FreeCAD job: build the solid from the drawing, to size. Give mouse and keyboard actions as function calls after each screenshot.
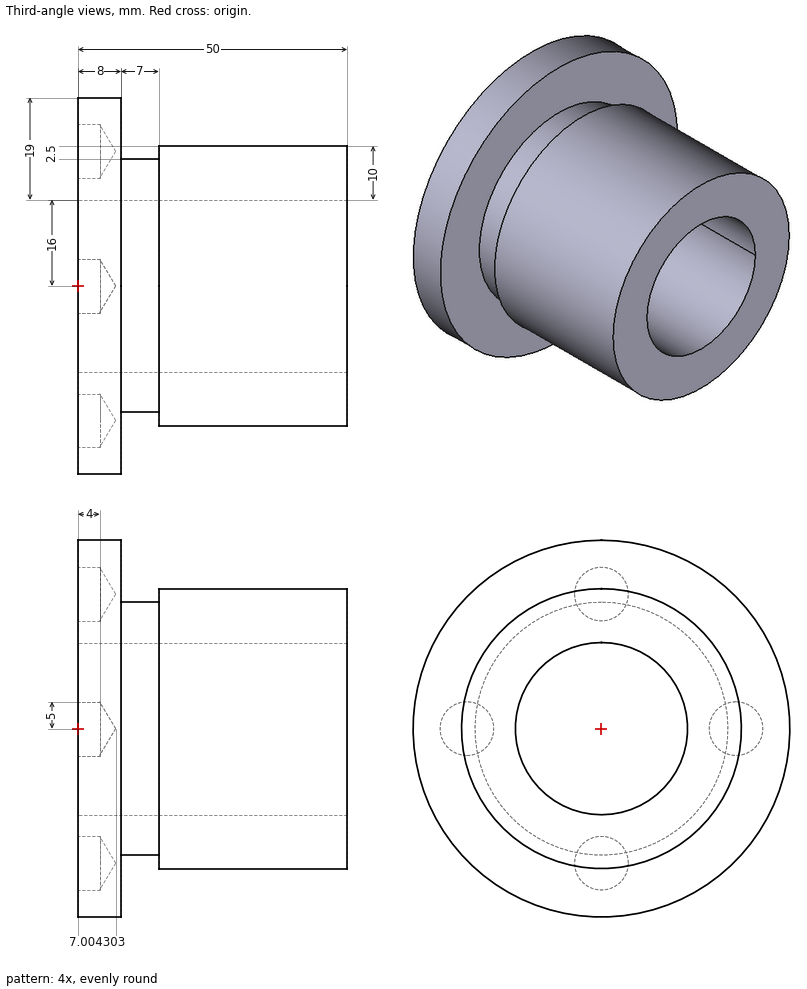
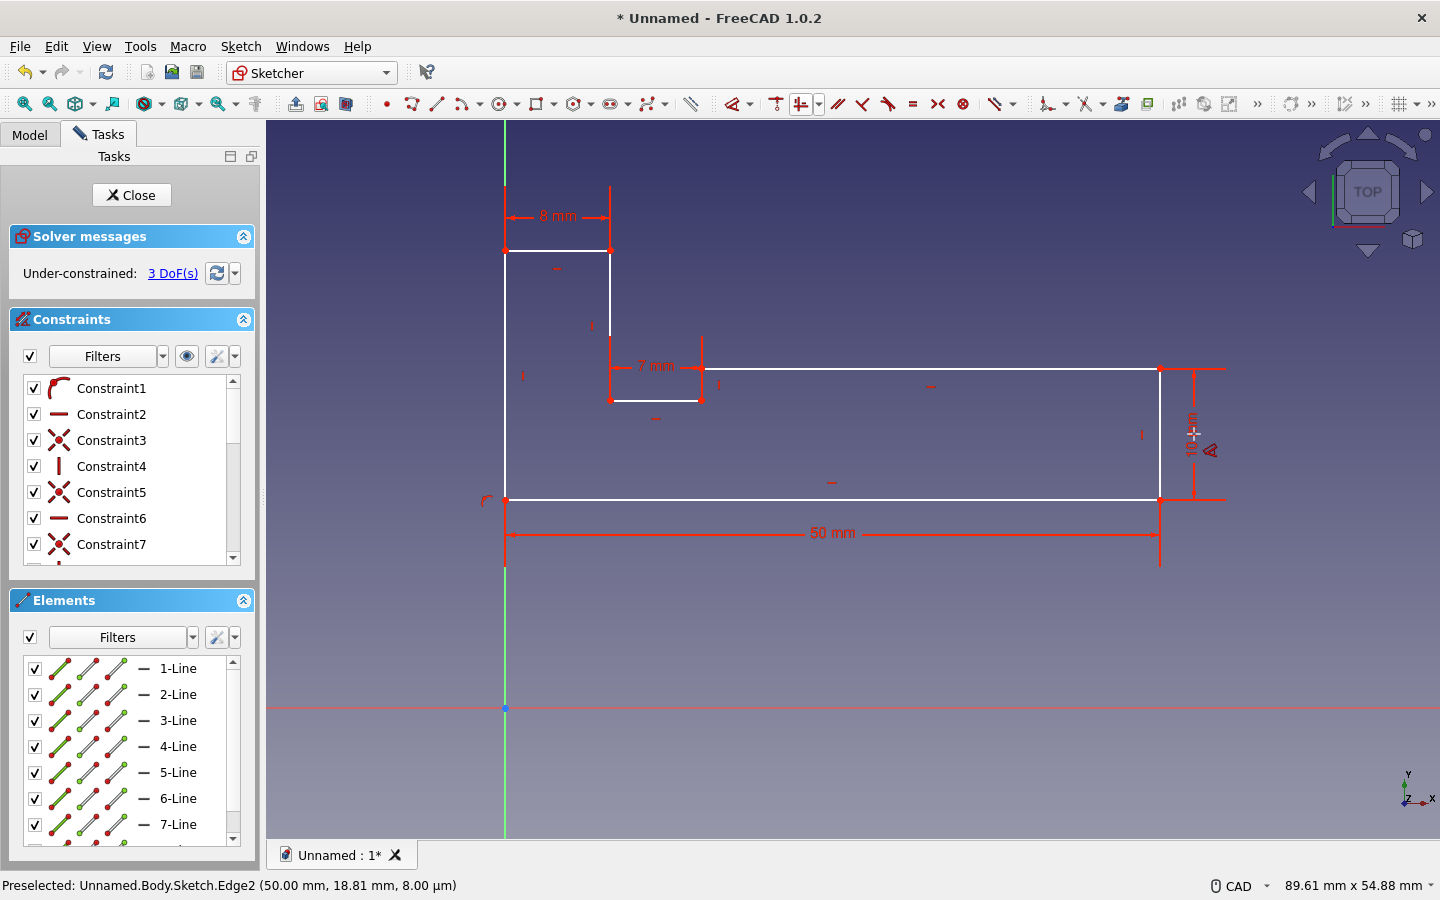
click(505, 326)
click(471, 376)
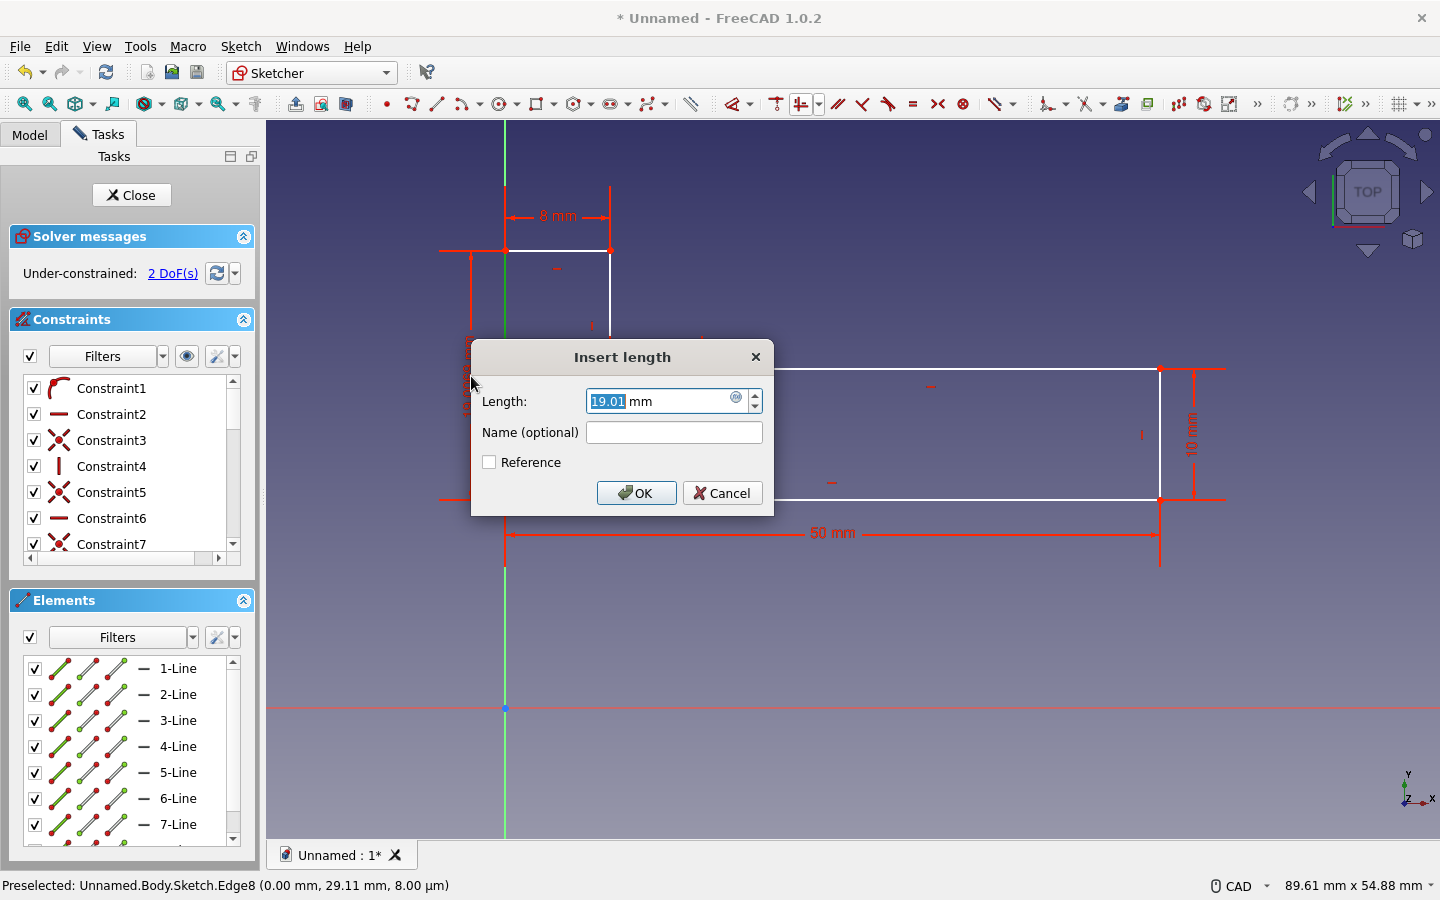
text(19)
key(Return)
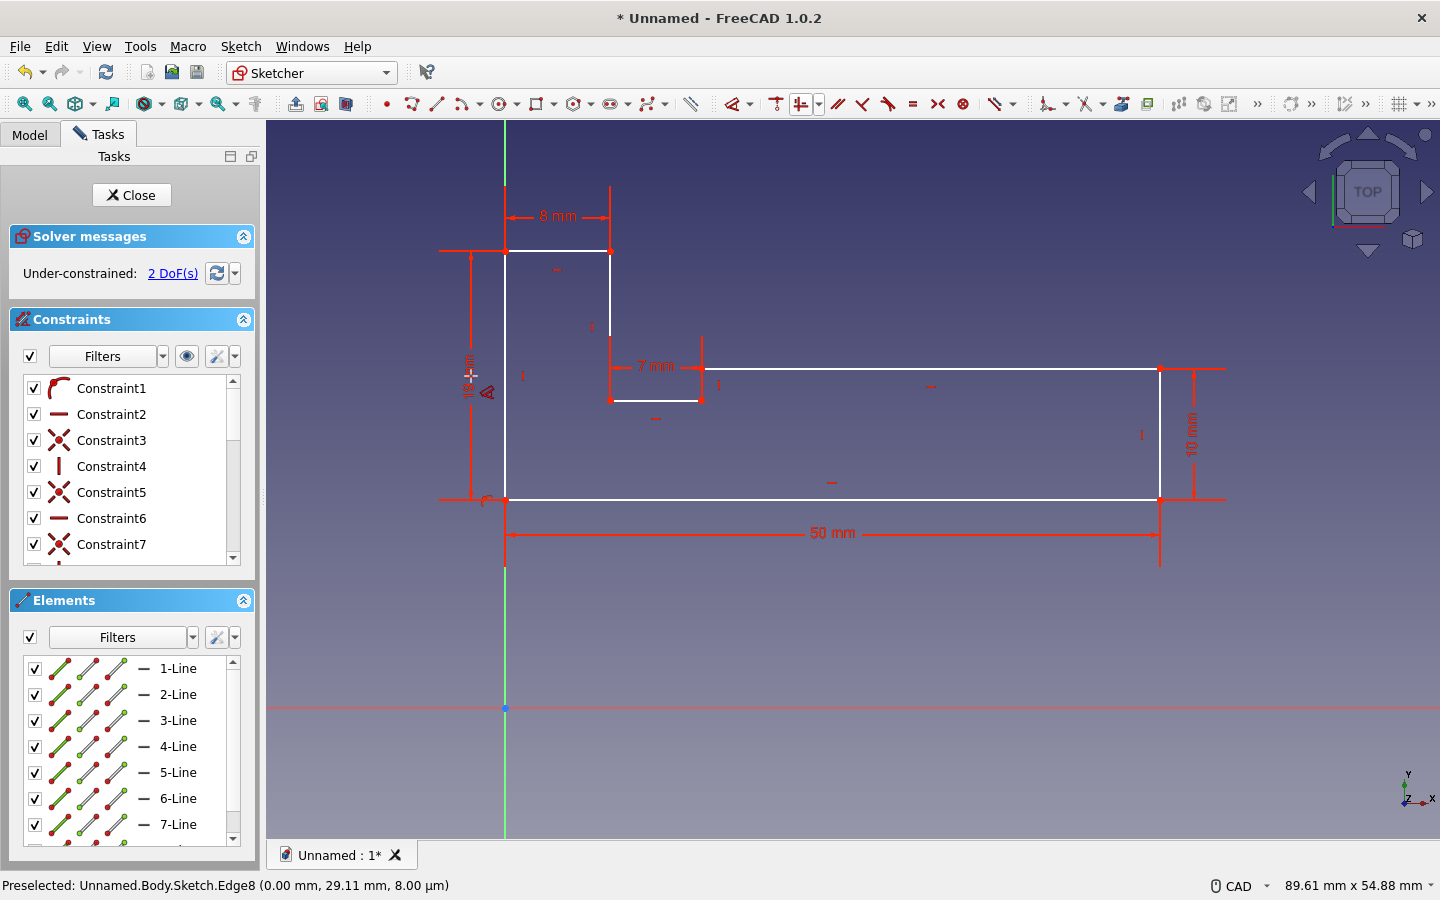
scroll(702, 379, up, 2)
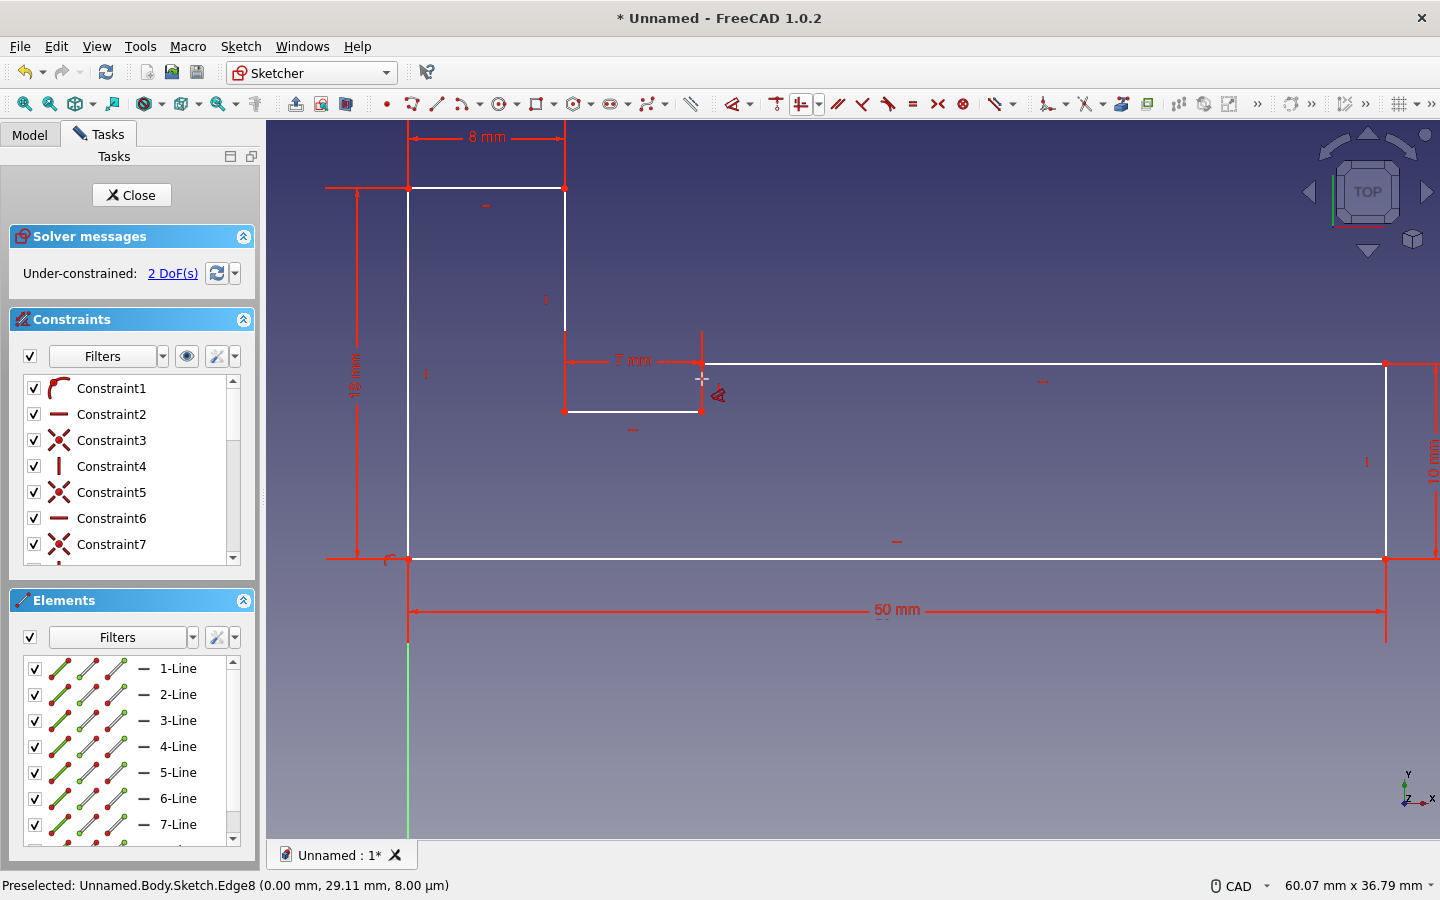
click(702, 378)
click(668, 388)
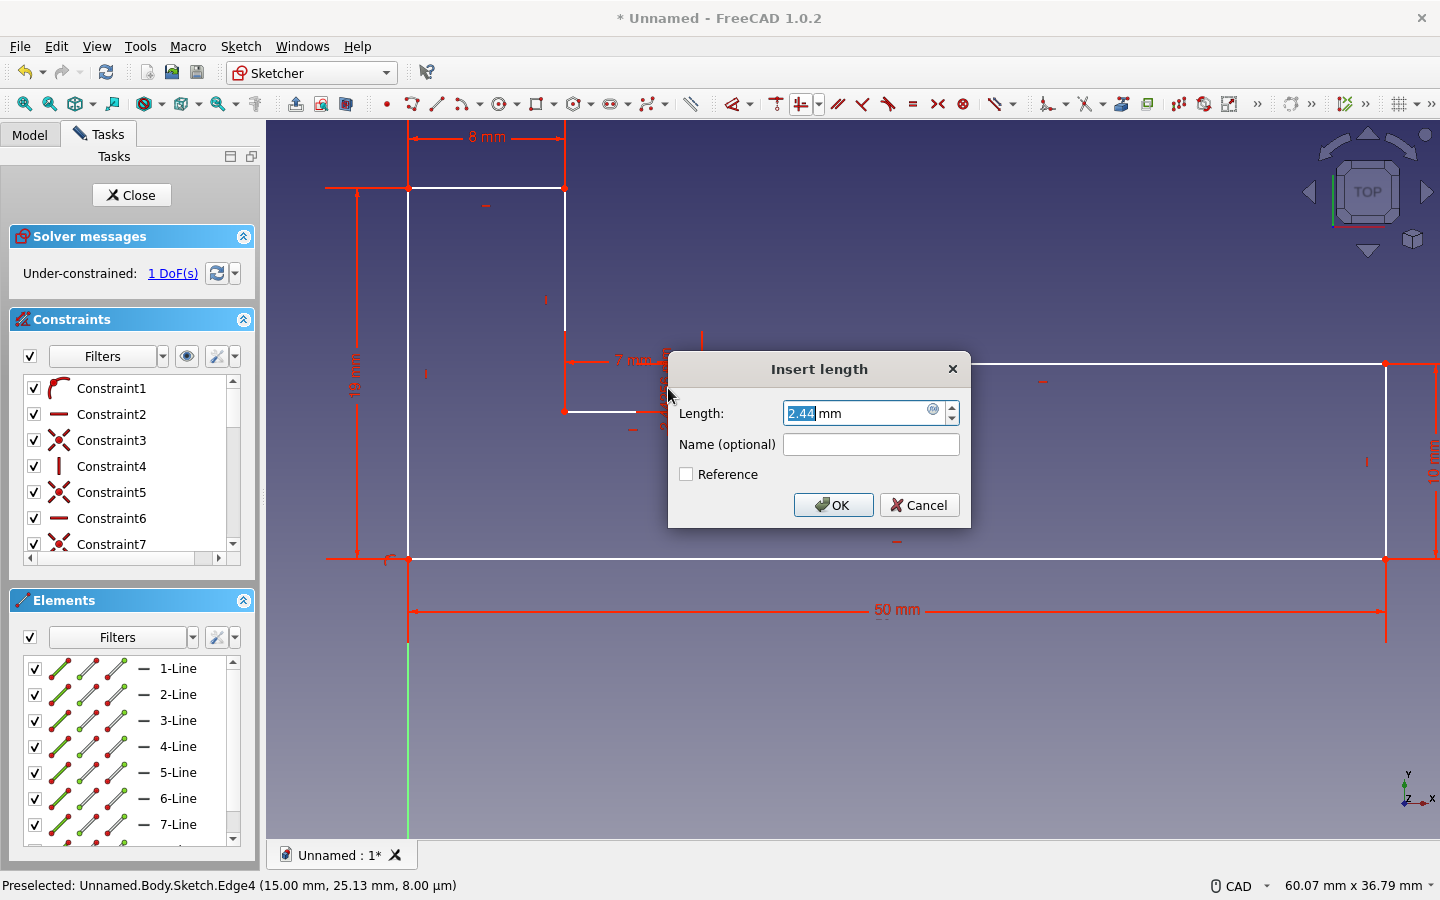
text(2.5)
key(Return)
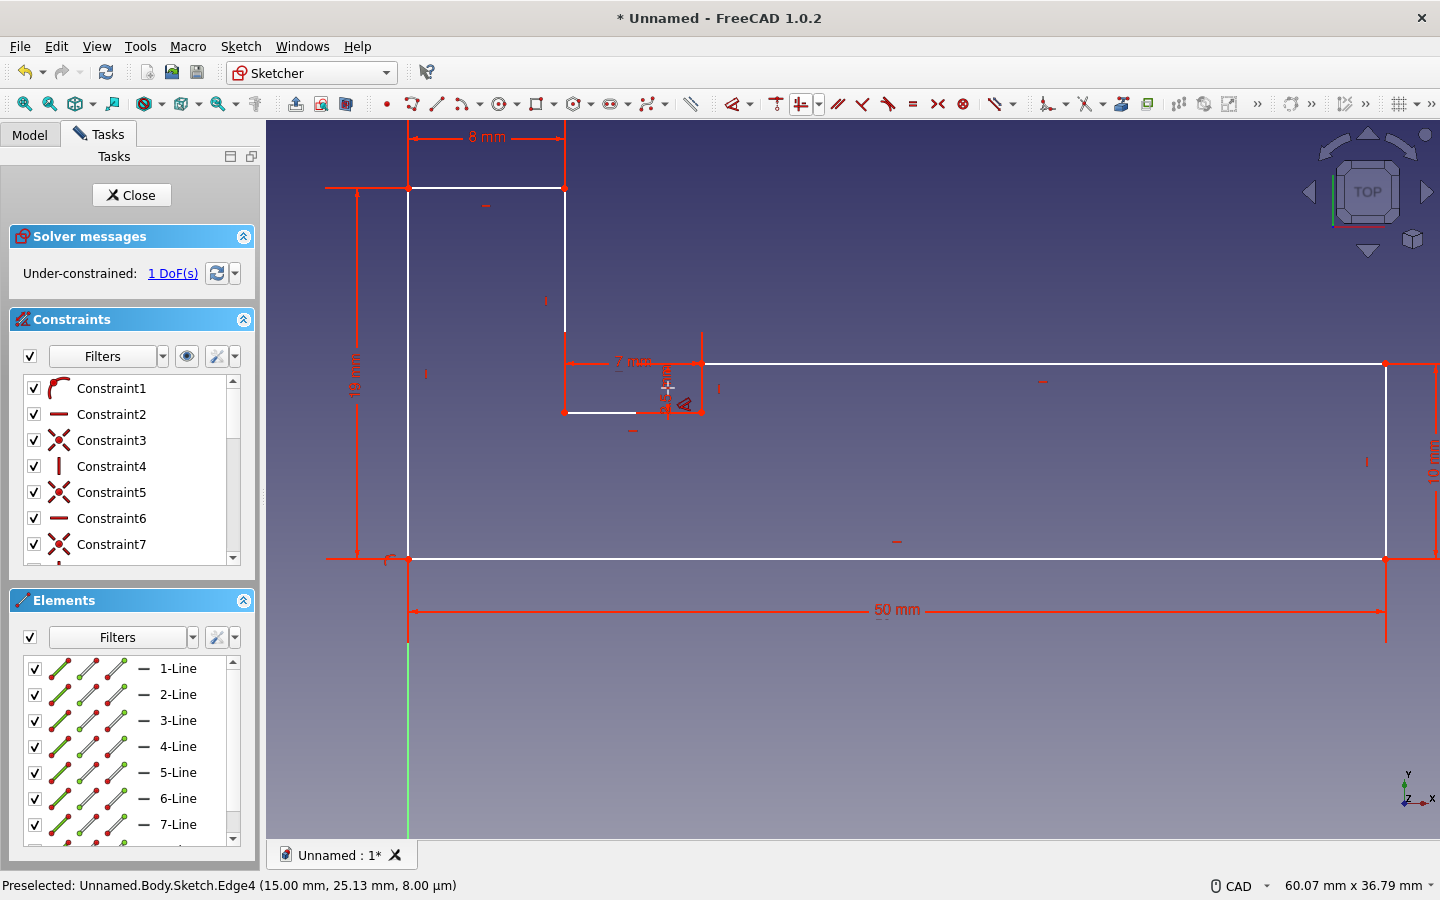
click(408, 559)
click(374, 685)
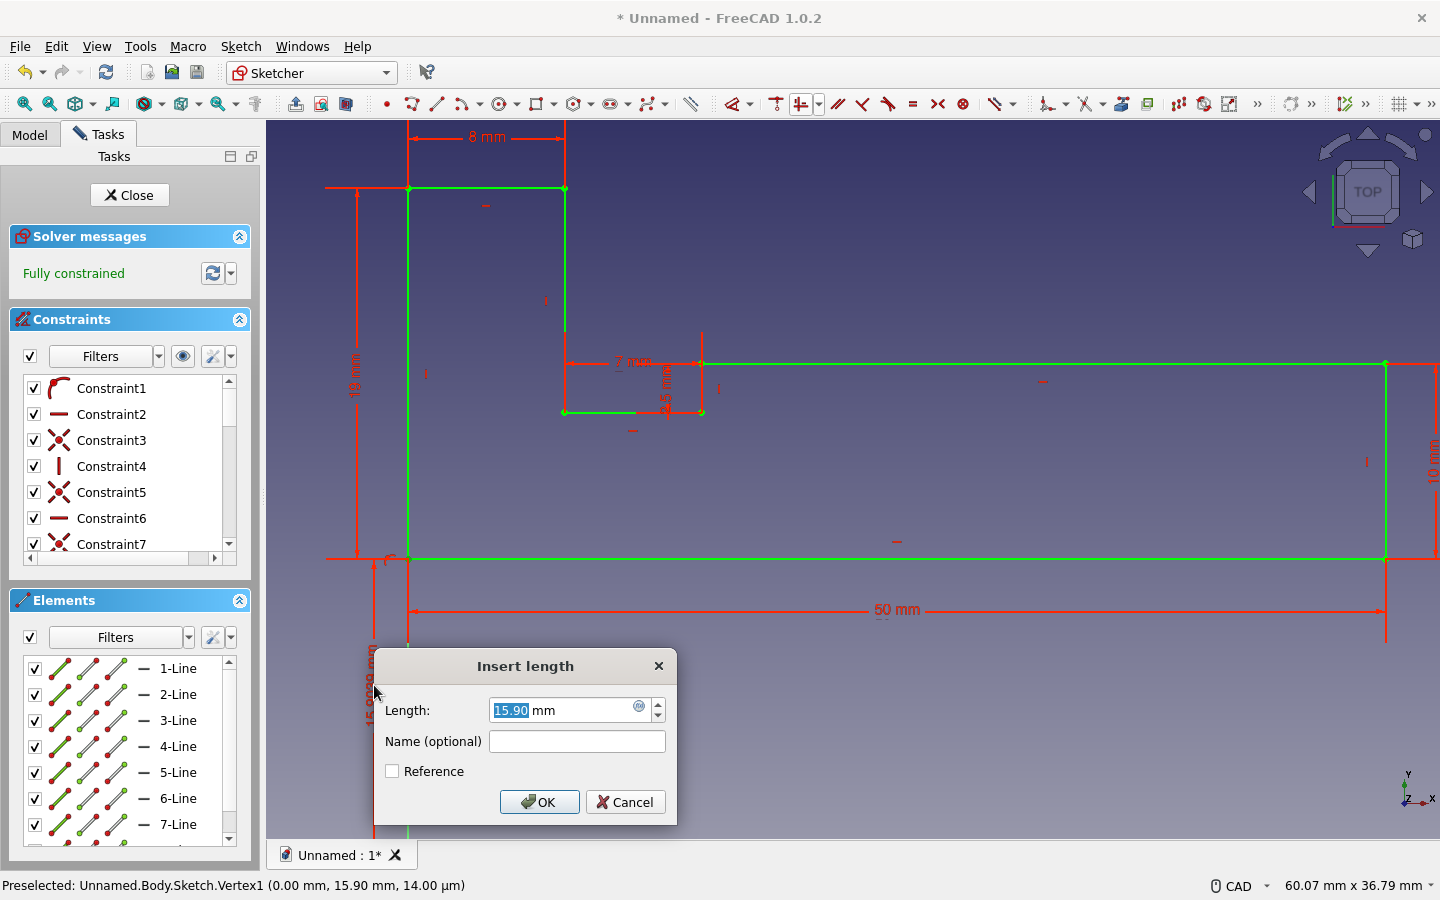
text(16)
key(Return)
key(Escape)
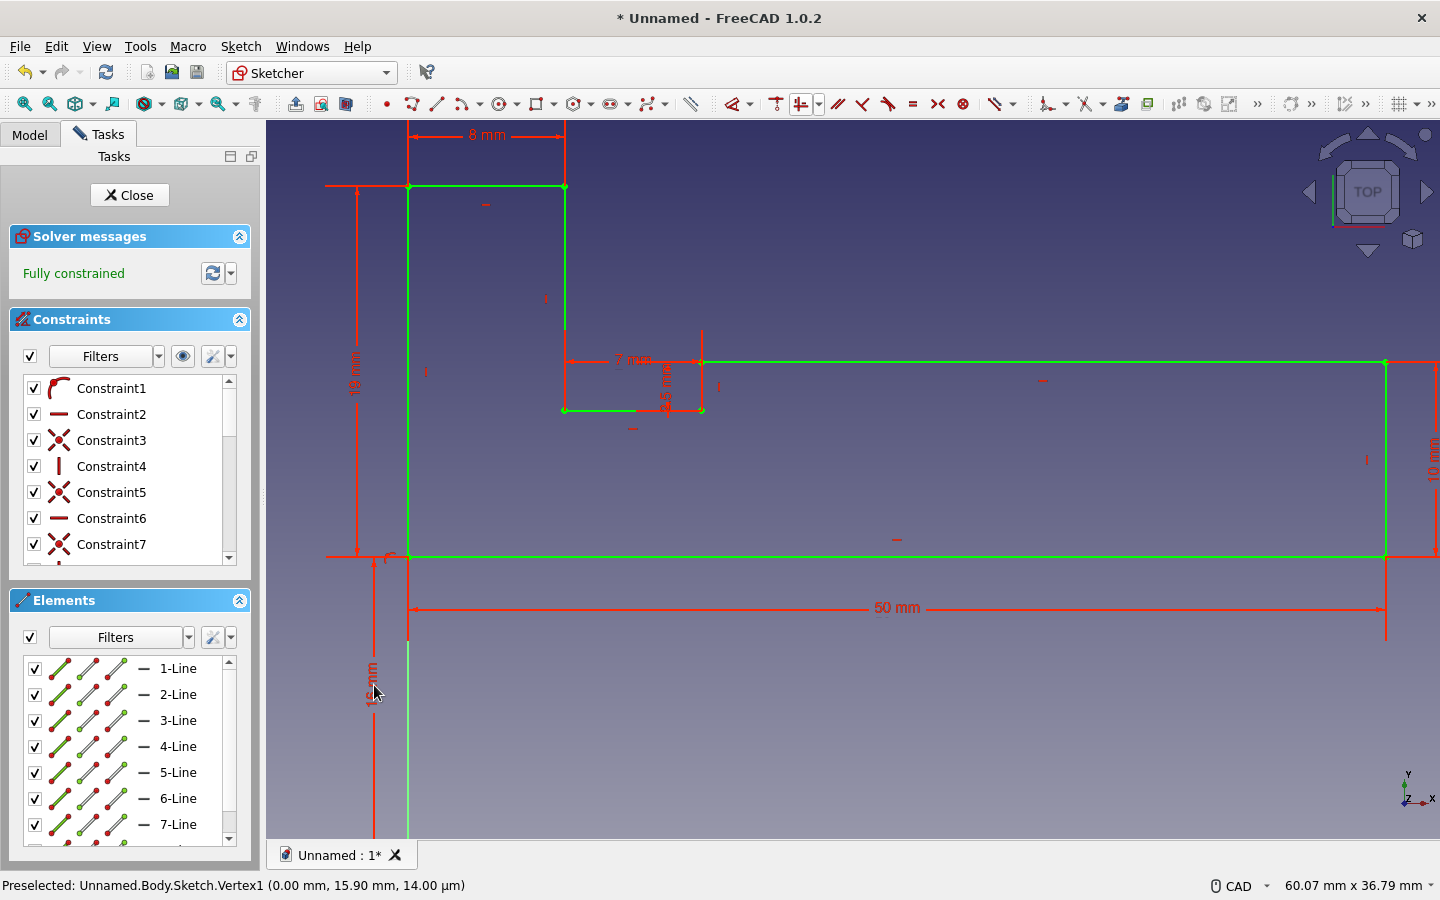
click(130, 195)